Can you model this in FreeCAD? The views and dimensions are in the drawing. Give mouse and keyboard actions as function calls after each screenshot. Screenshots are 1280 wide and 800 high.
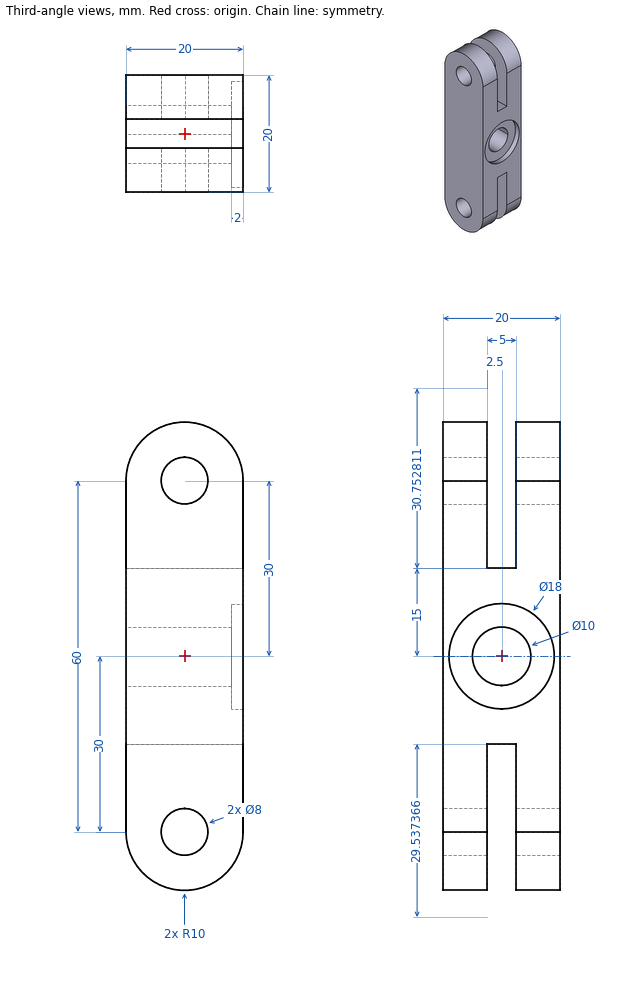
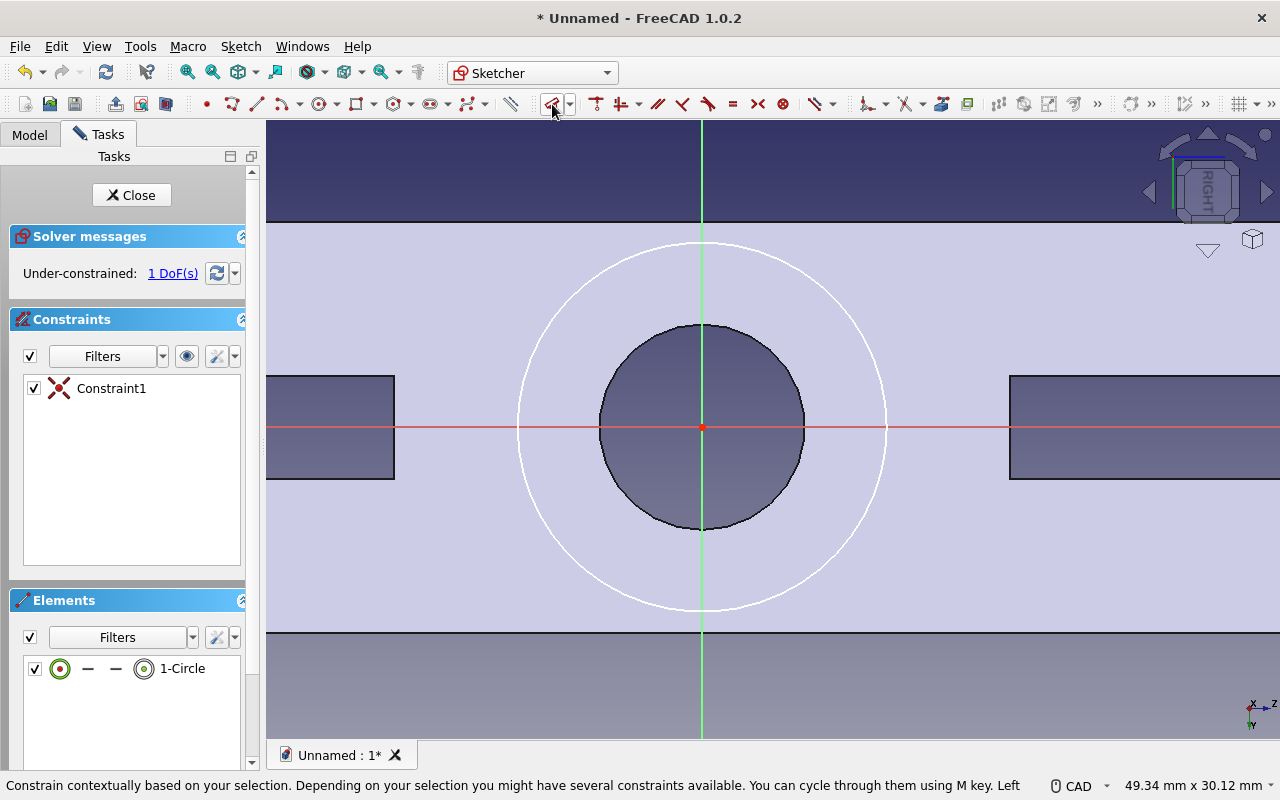
click(832, 296)
click(855, 273)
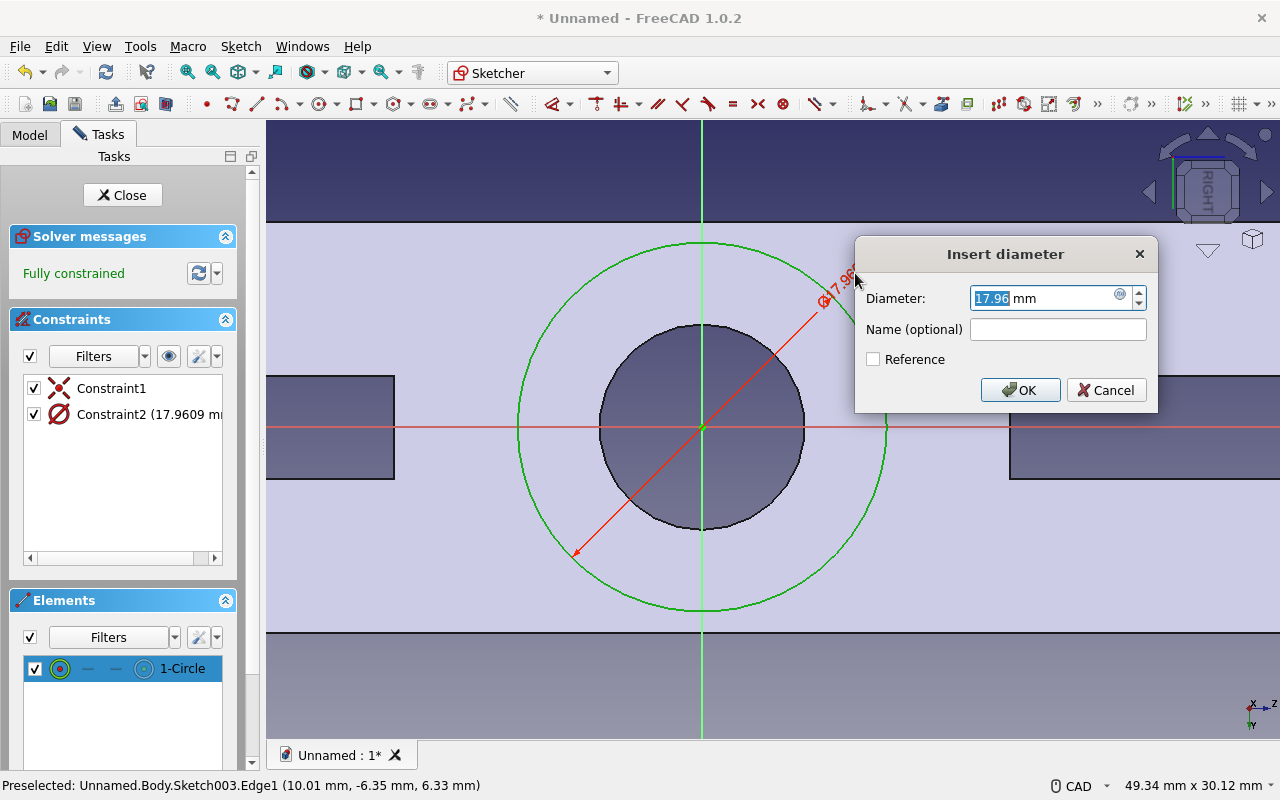
text(18)
key(Return)
key(Escape)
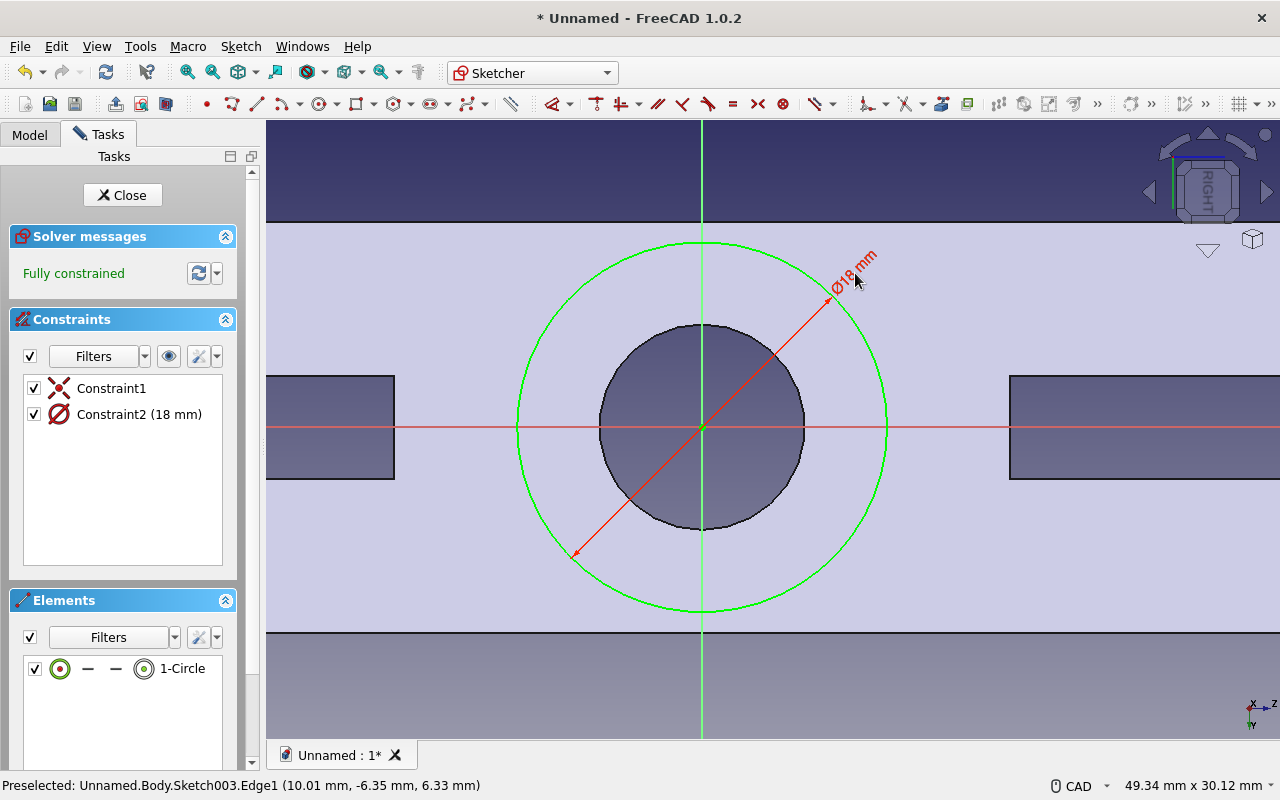
click(123, 195)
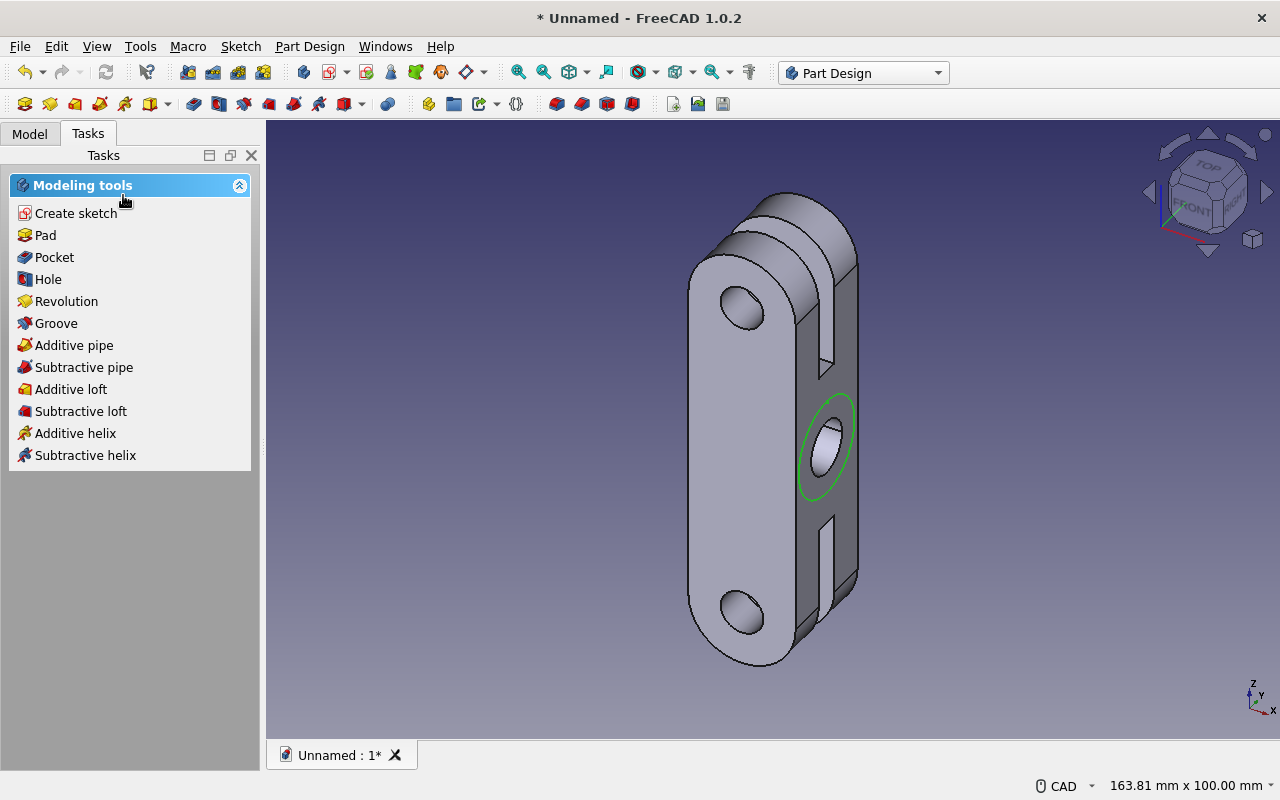
click(194, 104)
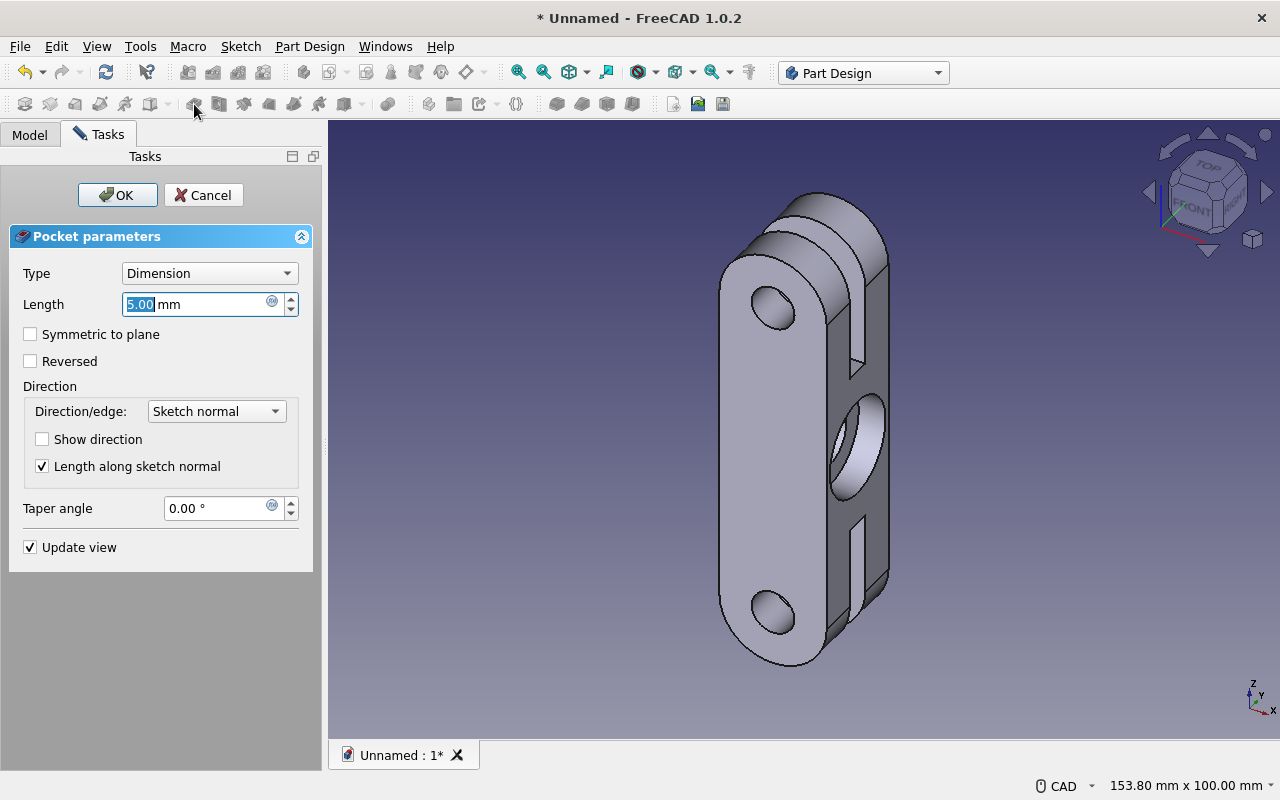
text(2)
key(Tab)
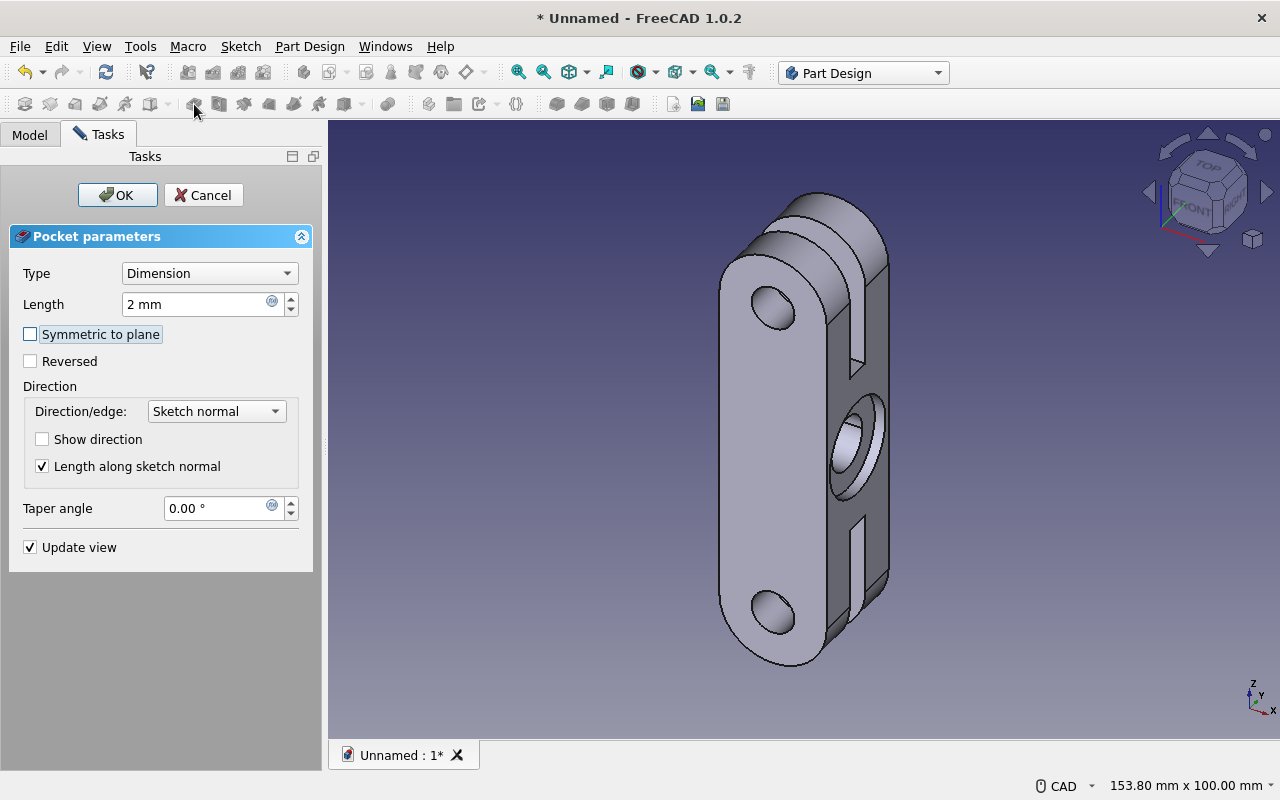
click(118, 195)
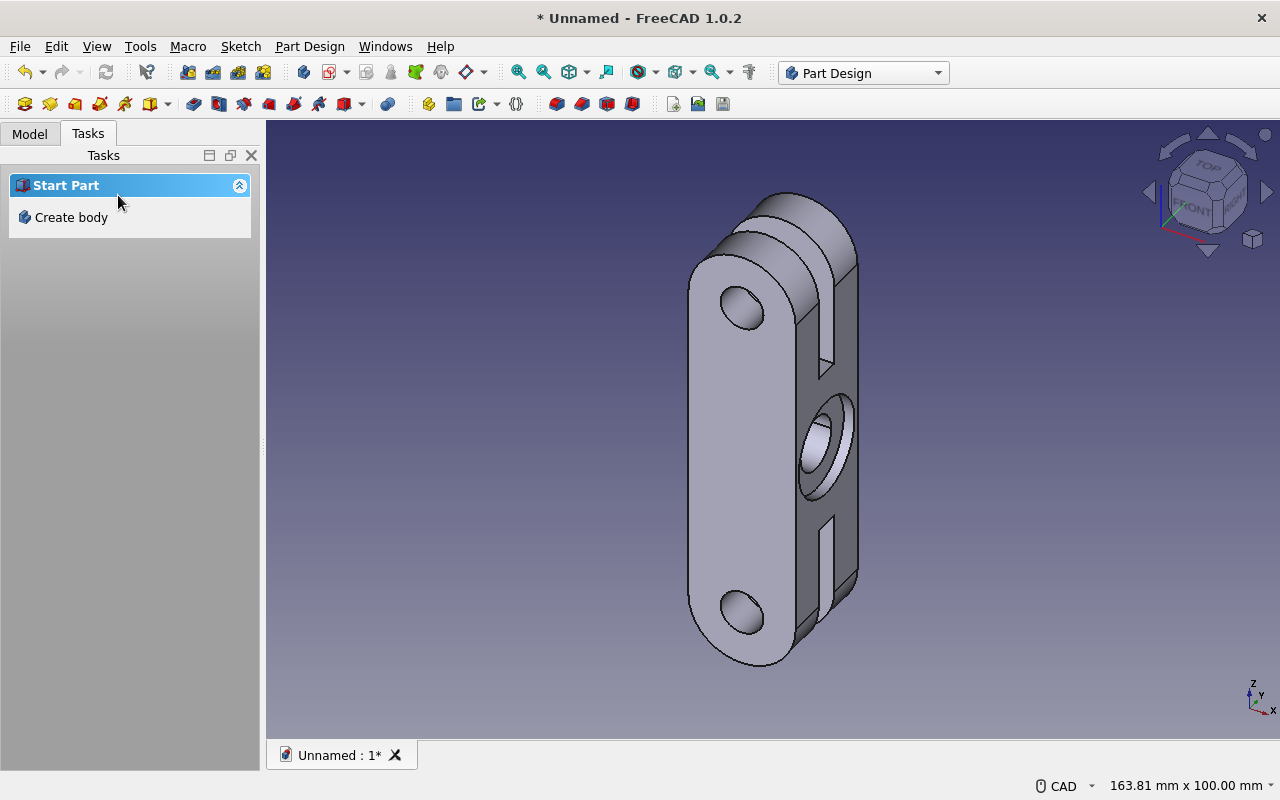
key(0)